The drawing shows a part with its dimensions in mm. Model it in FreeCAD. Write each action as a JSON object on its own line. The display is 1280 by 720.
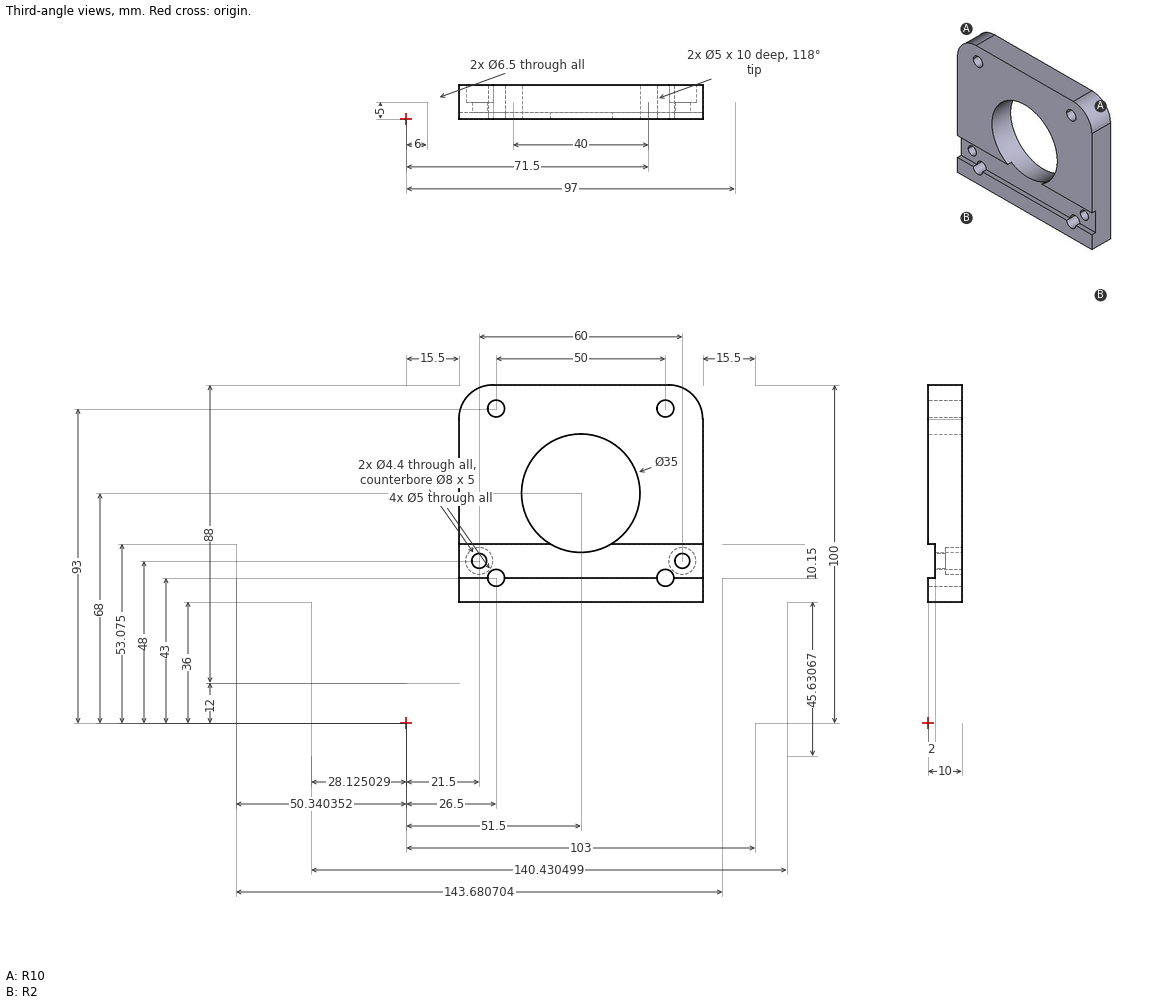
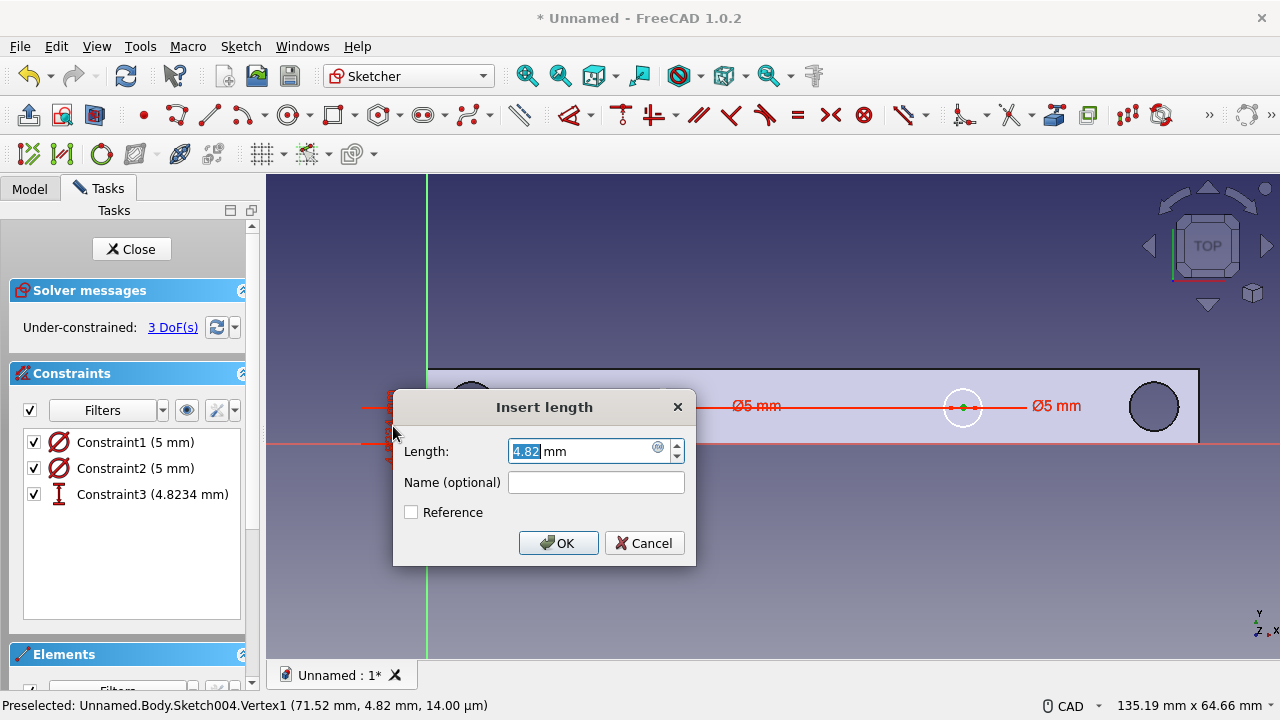
{"action": "type", "text": "5"}
{"action": "key", "text": "Return"}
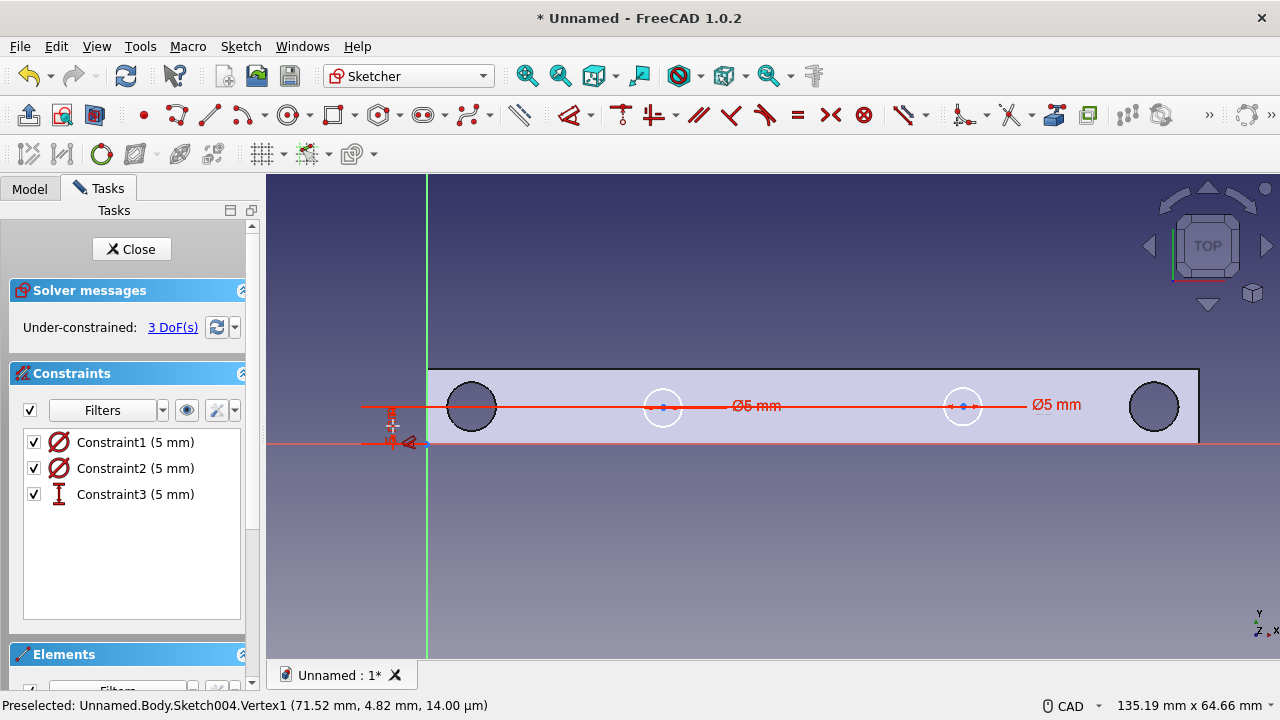
{"action": "left_click", "coordinate": [663, 408]}
{"action": "left_click", "coordinate": [697, 426]}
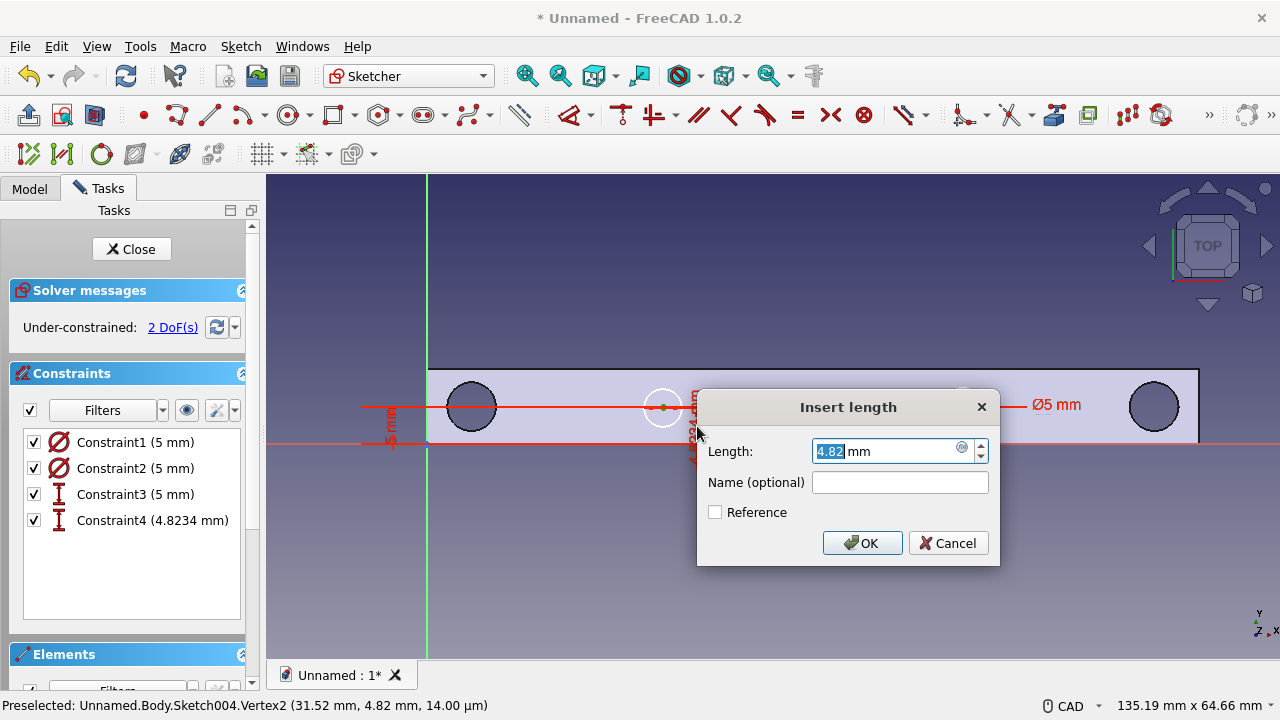
{"action": "type", "text": "5"}
{"action": "key", "text": "Return"}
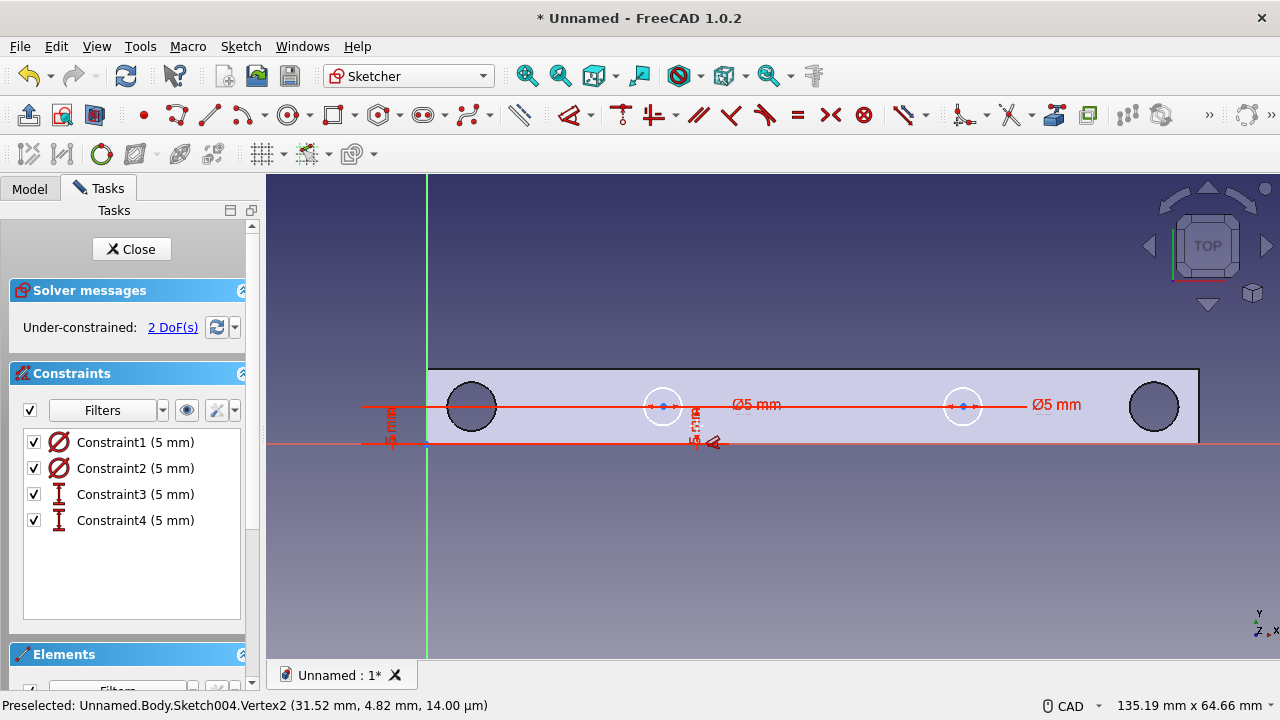
{"action": "left_click", "coordinate": [963, 407]}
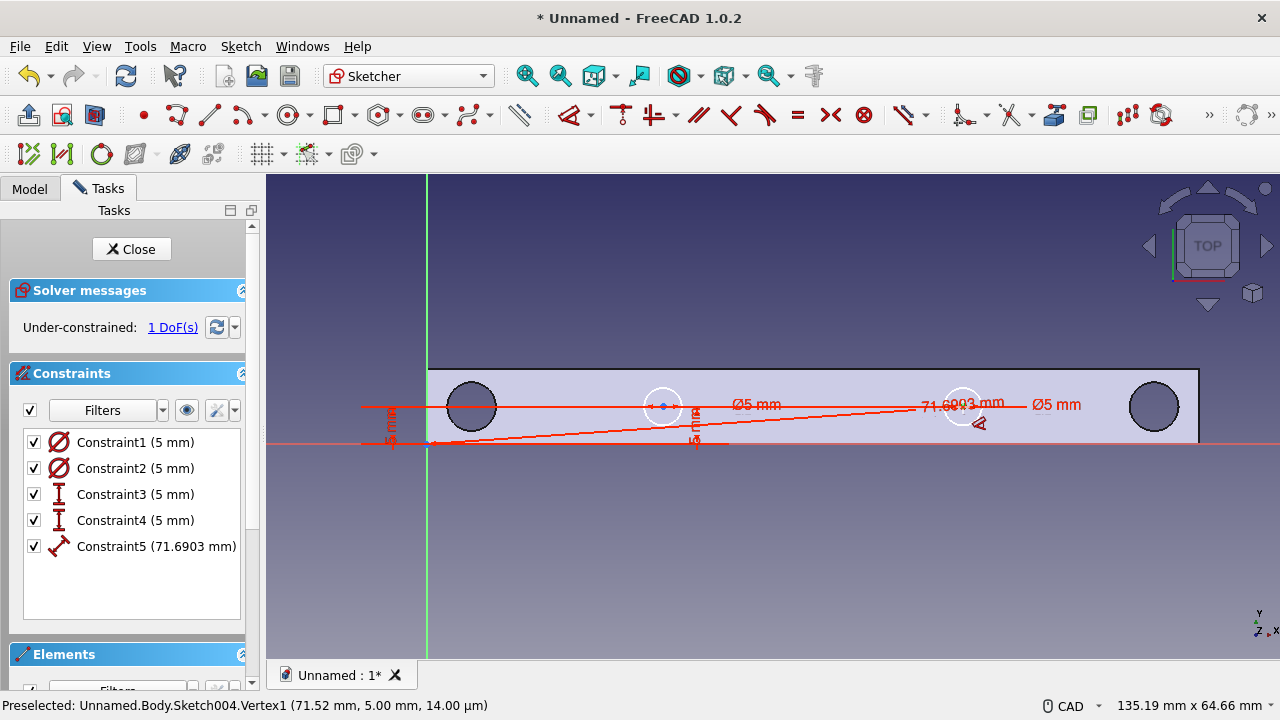
{"action": "left_click", "coordinate": [663, 407]}
{"action": "left_click", "coordinate": [813, 373]}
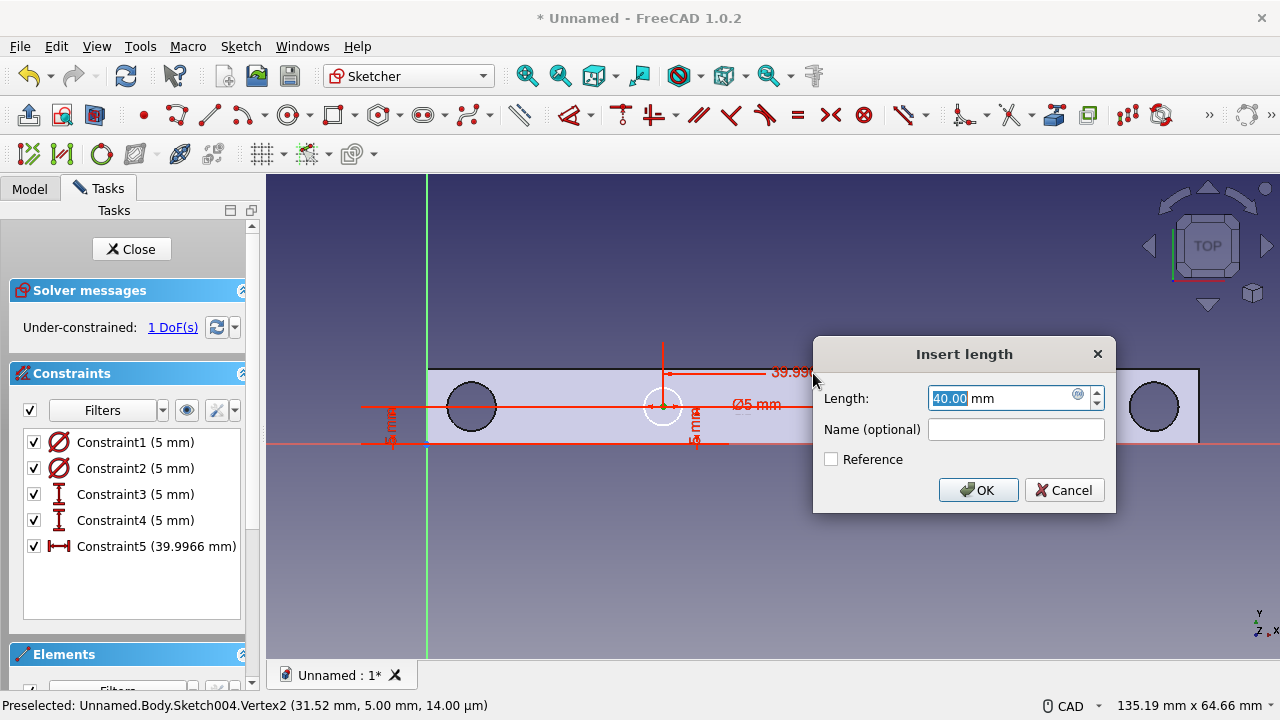
{"action": "type", "text": "40"}
{"action": "key", "text": "Return"}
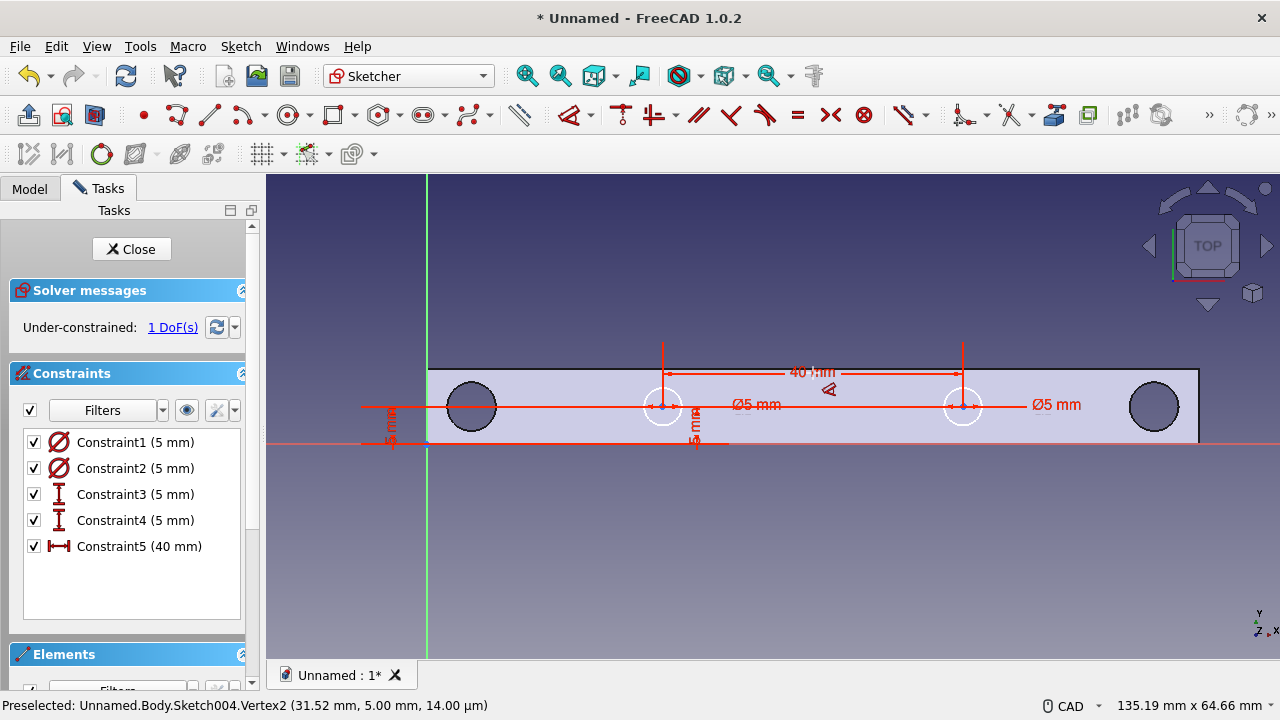
{"action": "left_click", "coordinate": [963, 407]}
{"action": "left_click", "coordinate": [695, 478]}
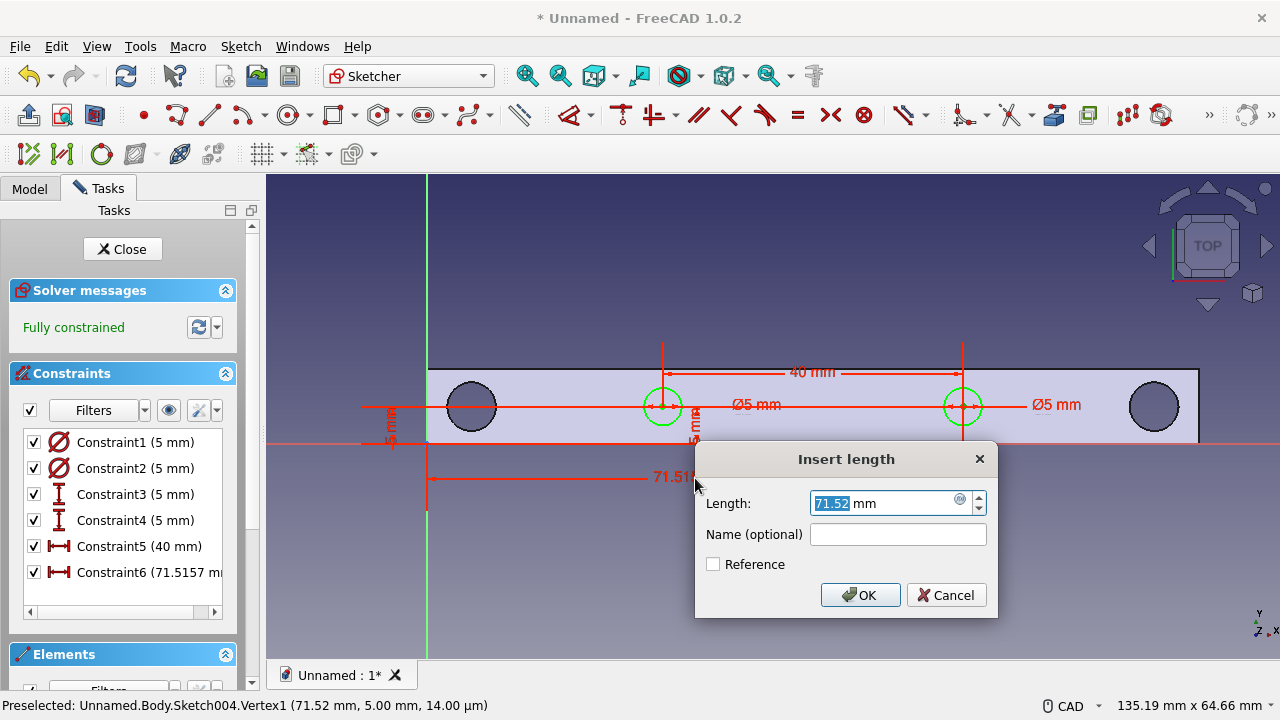
{"action": "type", "text": "71.5"}
{"action": "key", "text": "Return"}
{"action": "key", "text": "Escape"}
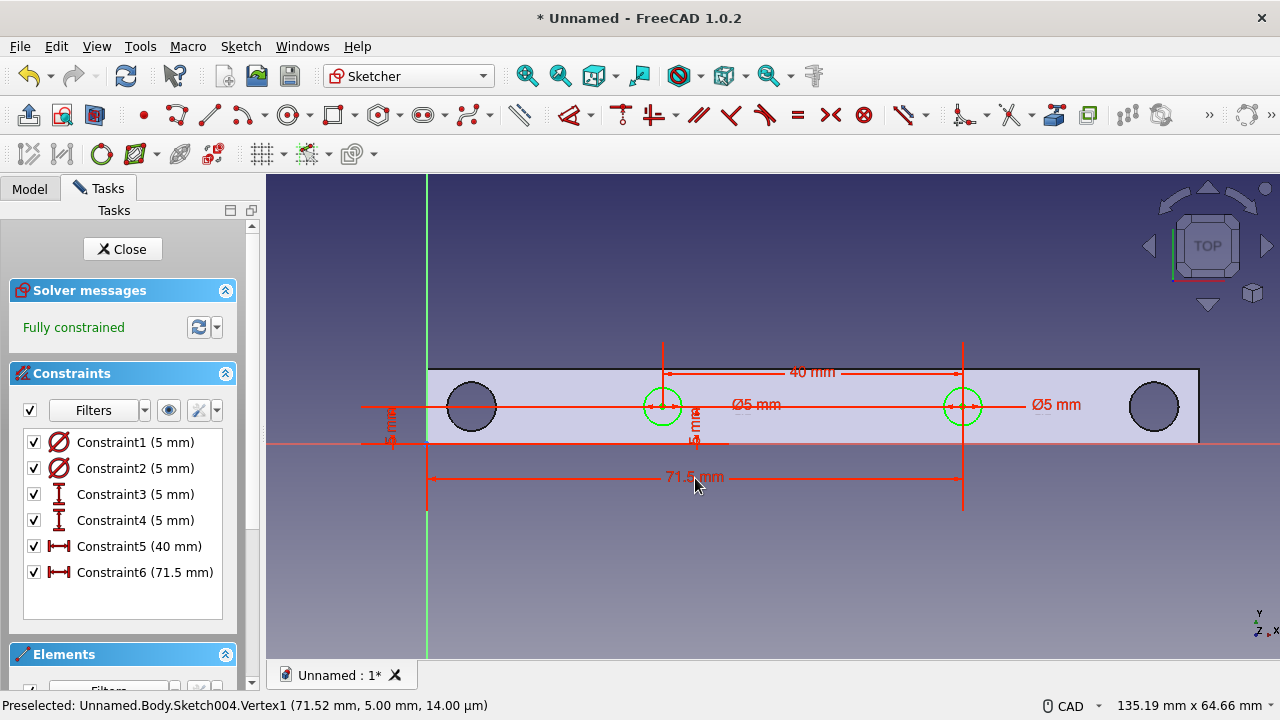
{"action": "left_click", "coordinate": [123, 249]}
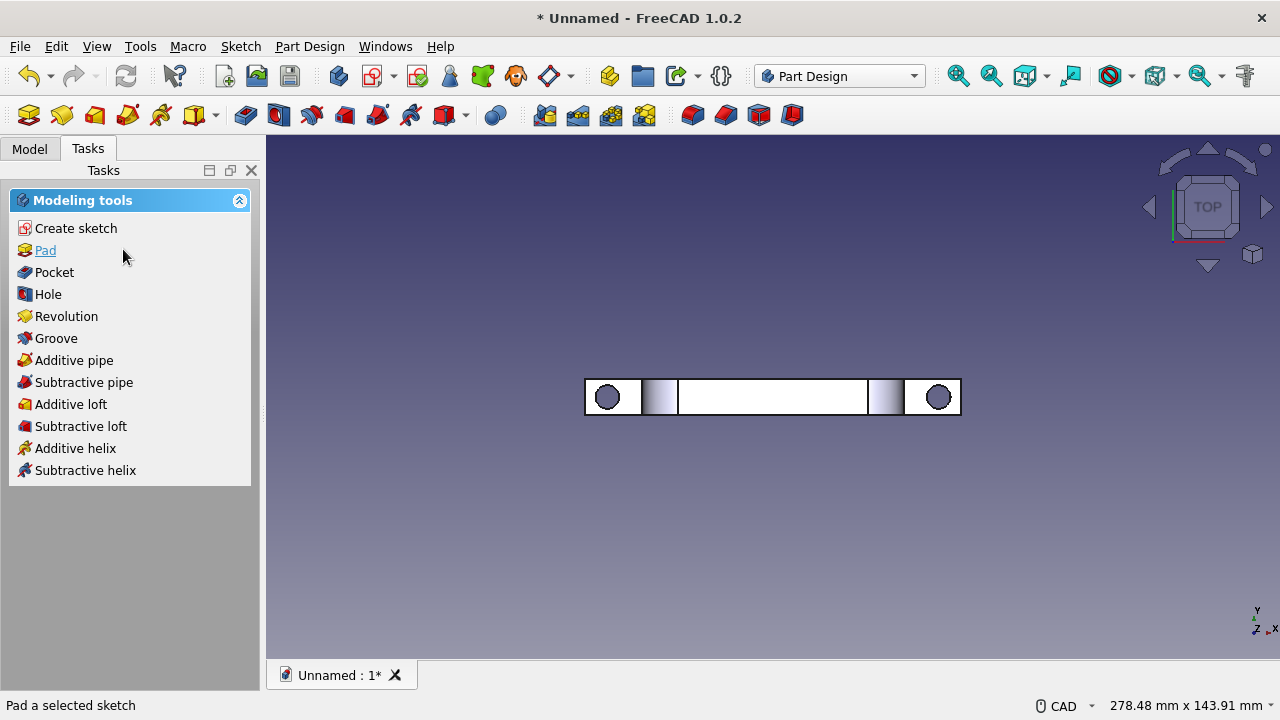
{"action": "left_click", "coordinate": [279, 116]}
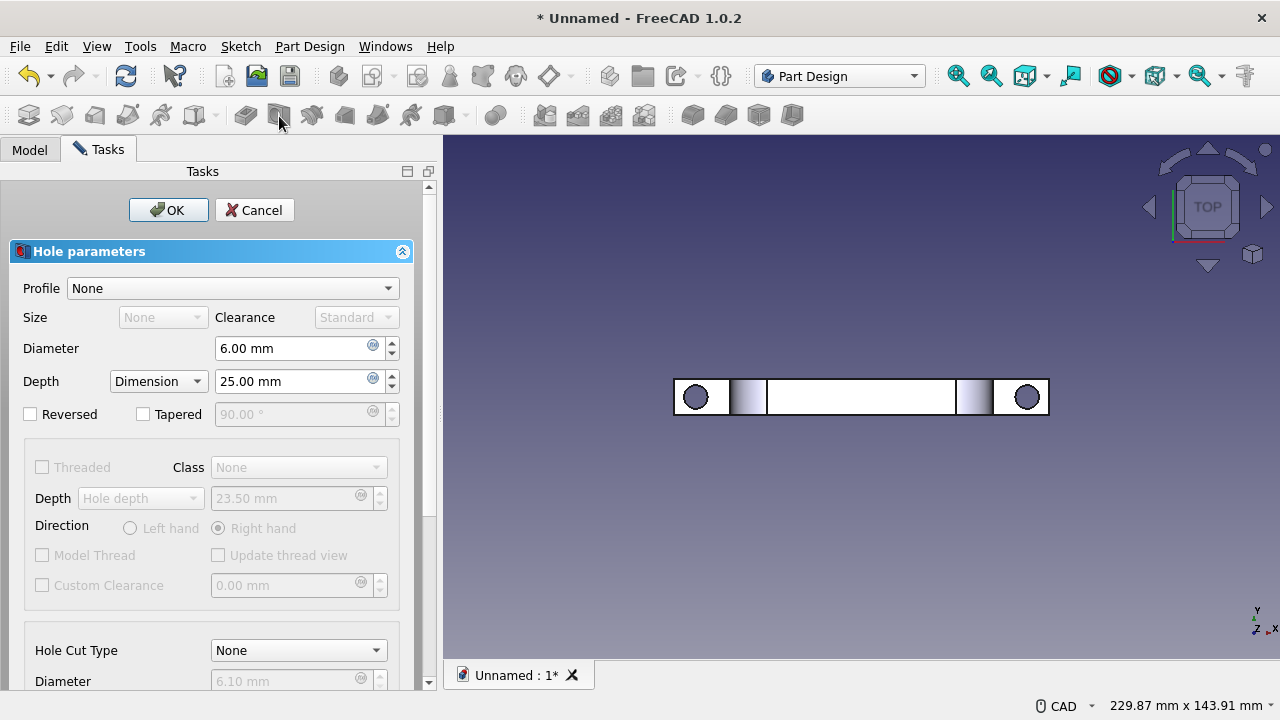
{"action": "triple_click", "coordinate": [300, 348]}